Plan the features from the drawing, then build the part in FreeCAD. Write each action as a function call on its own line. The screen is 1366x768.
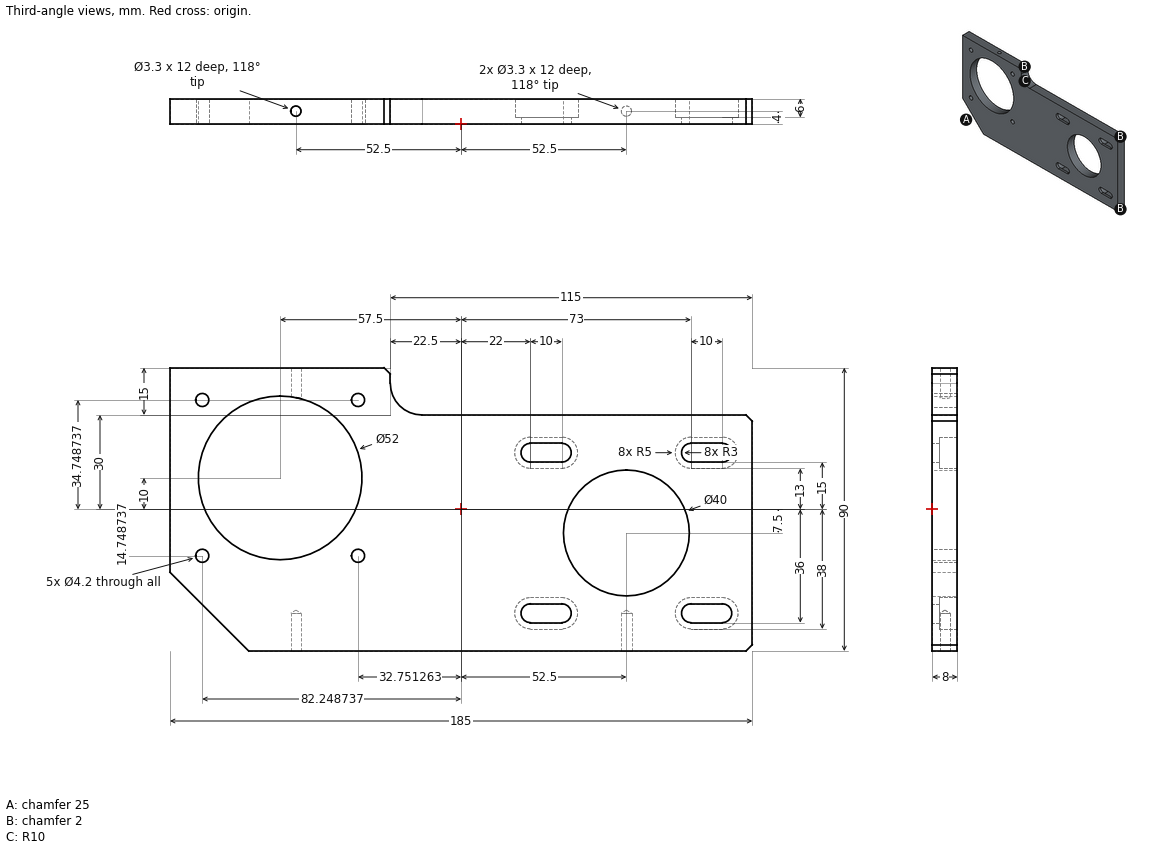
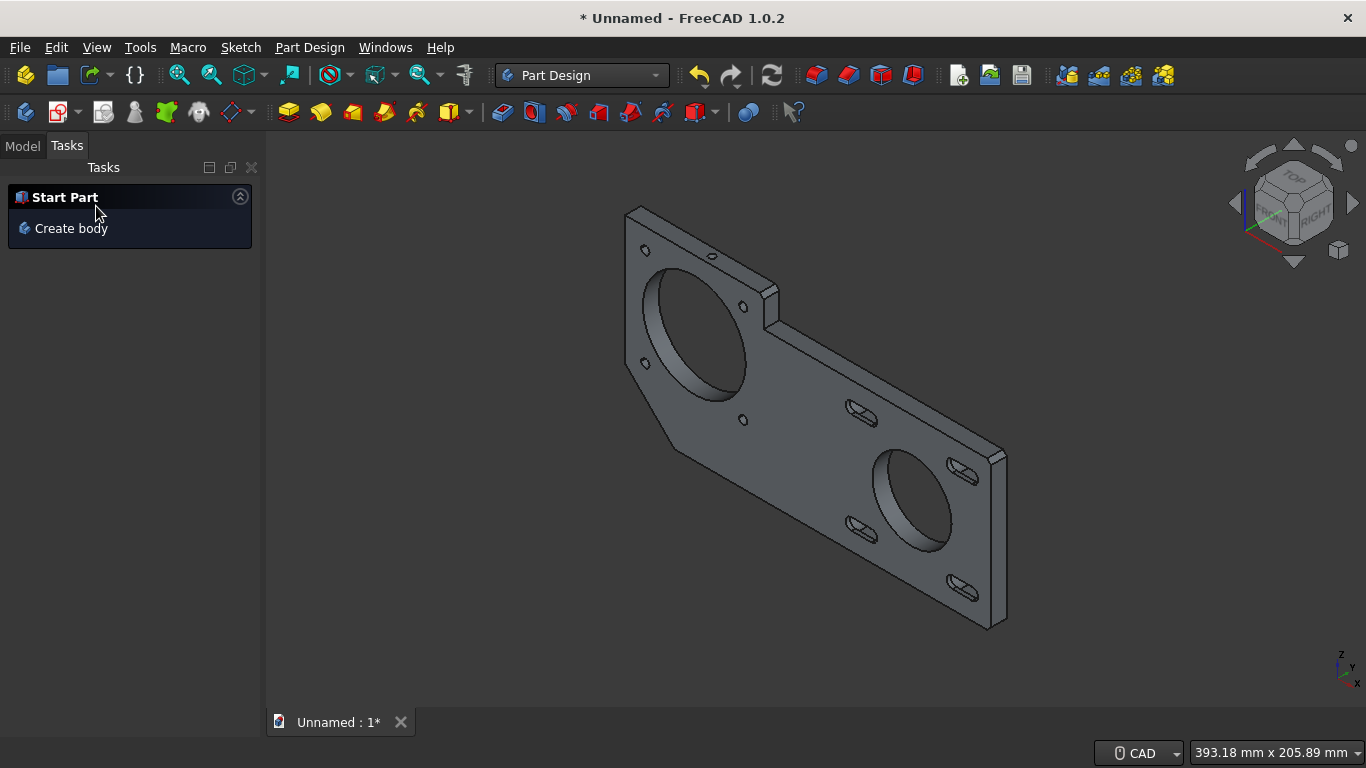
key(2)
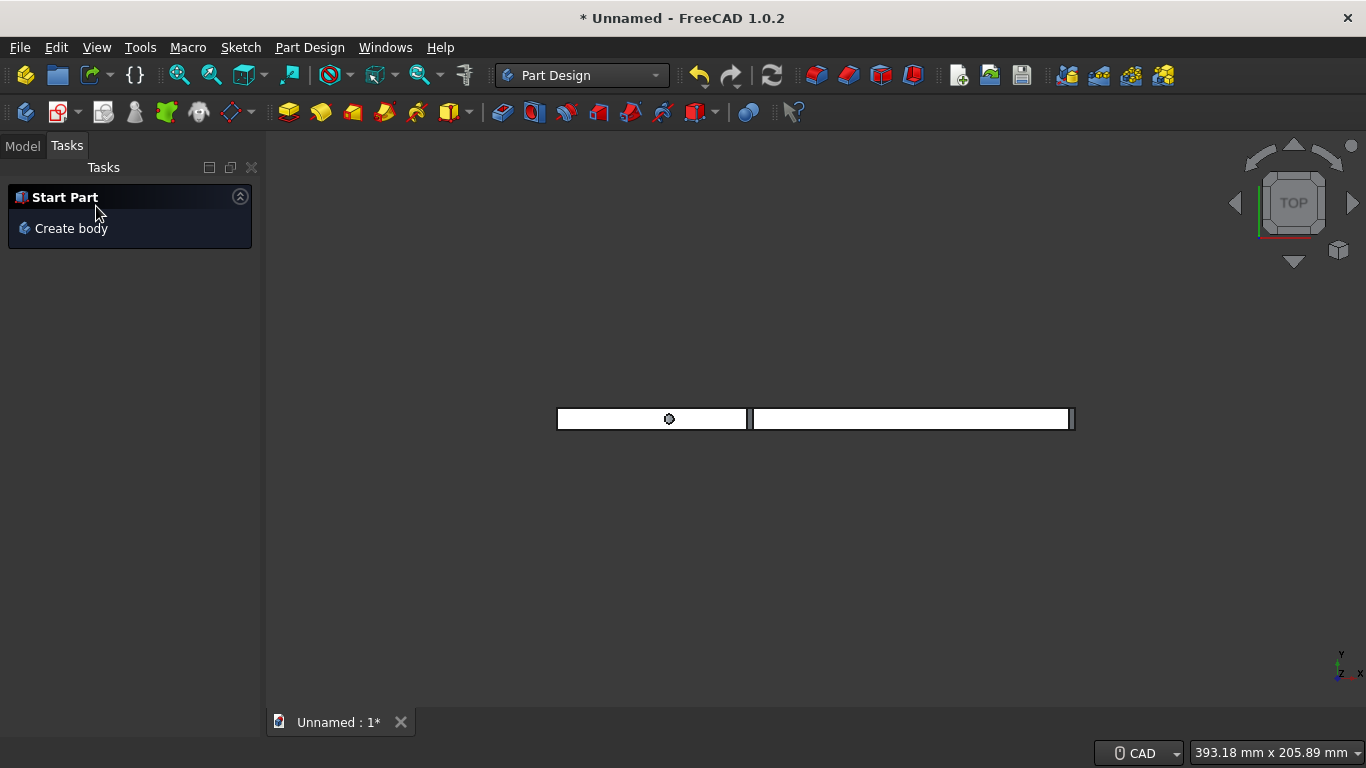
key(0)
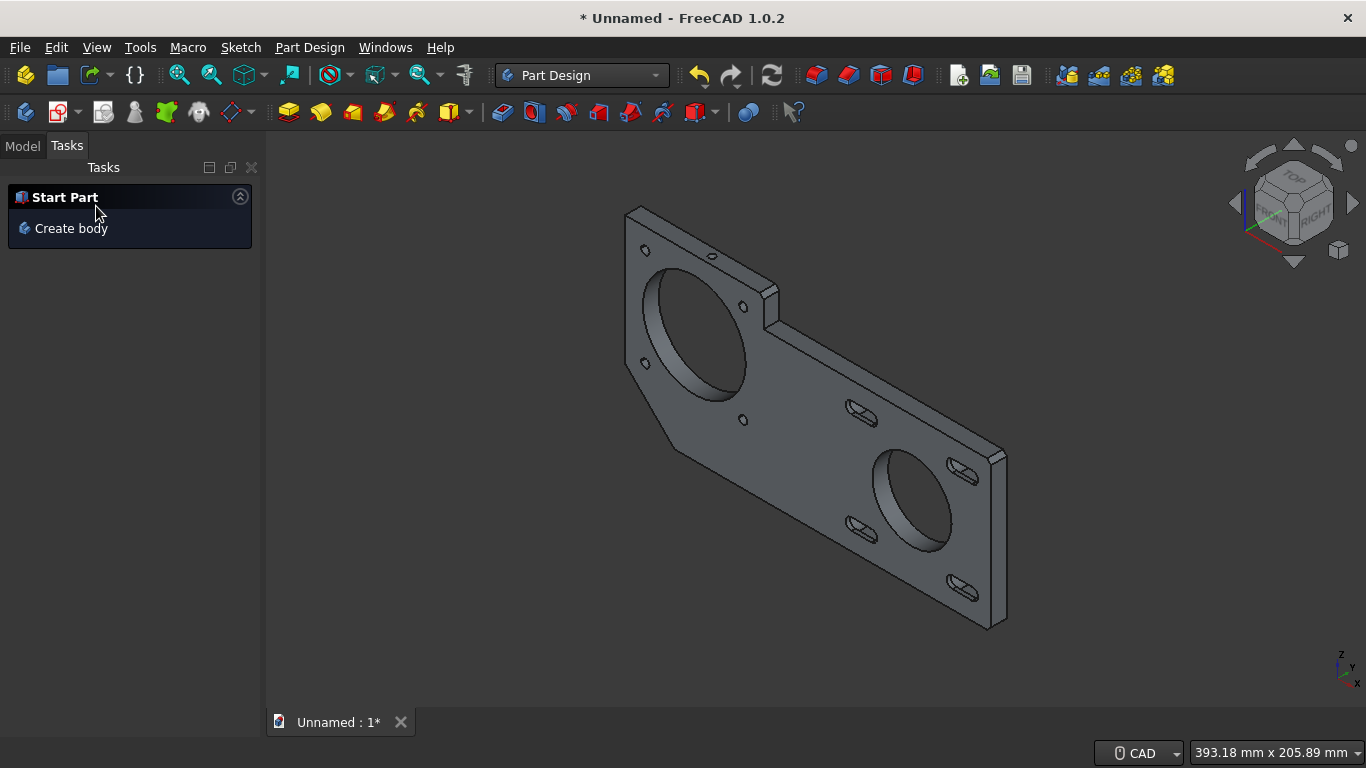
key(1)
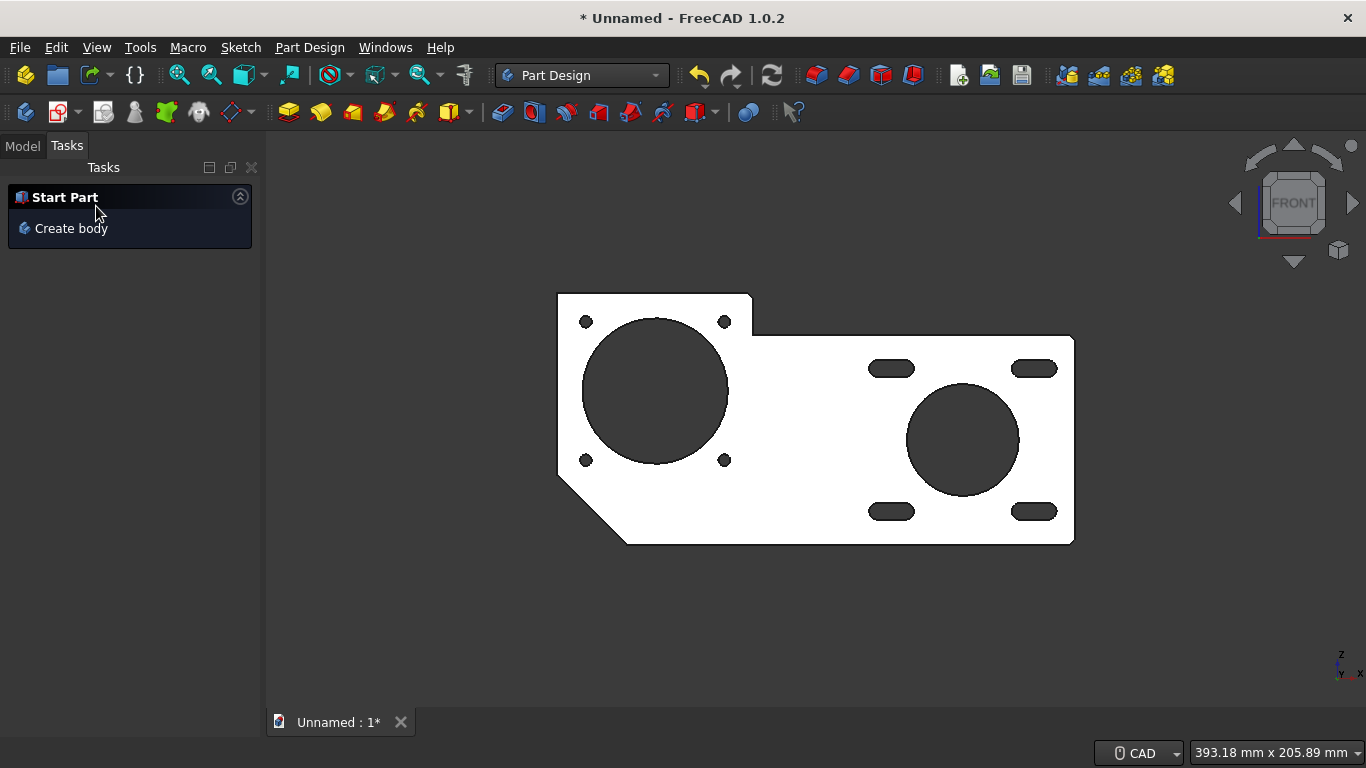
key(3)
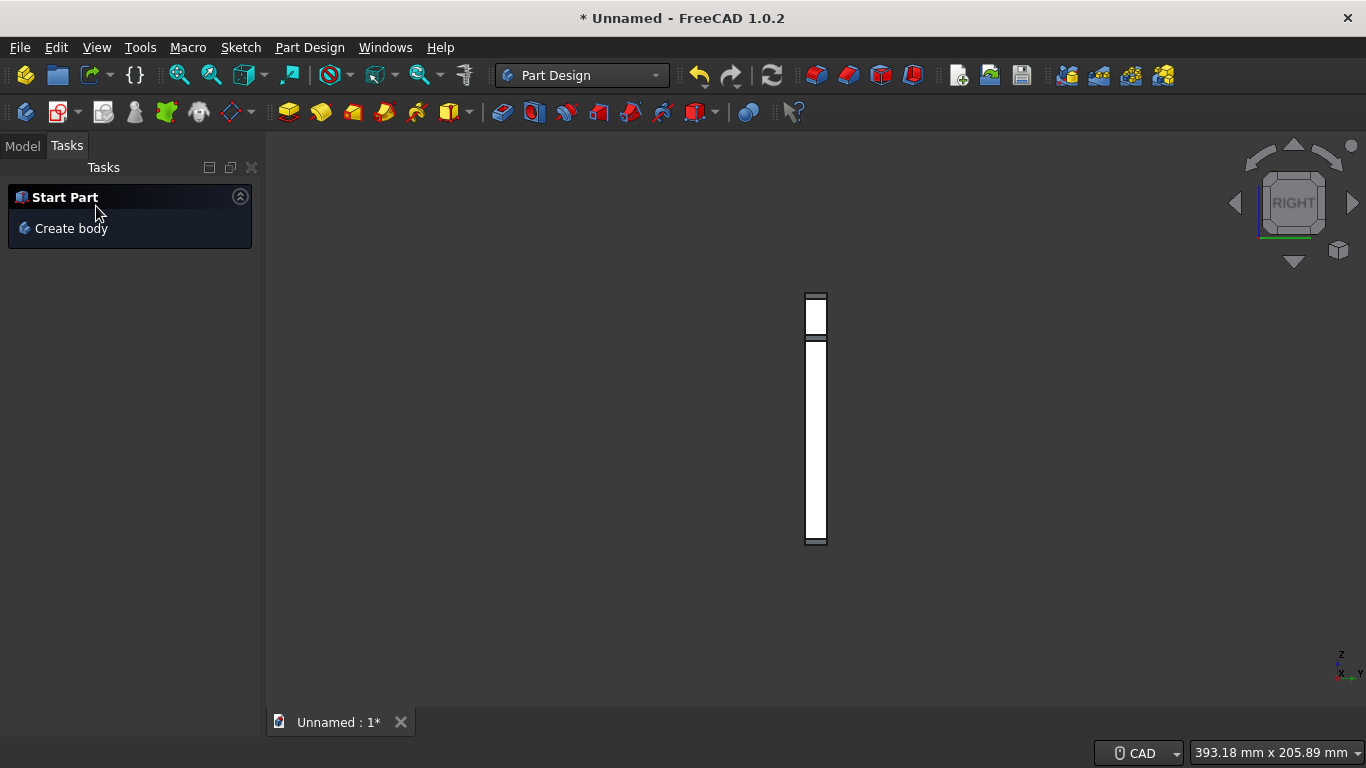
click(180, 76)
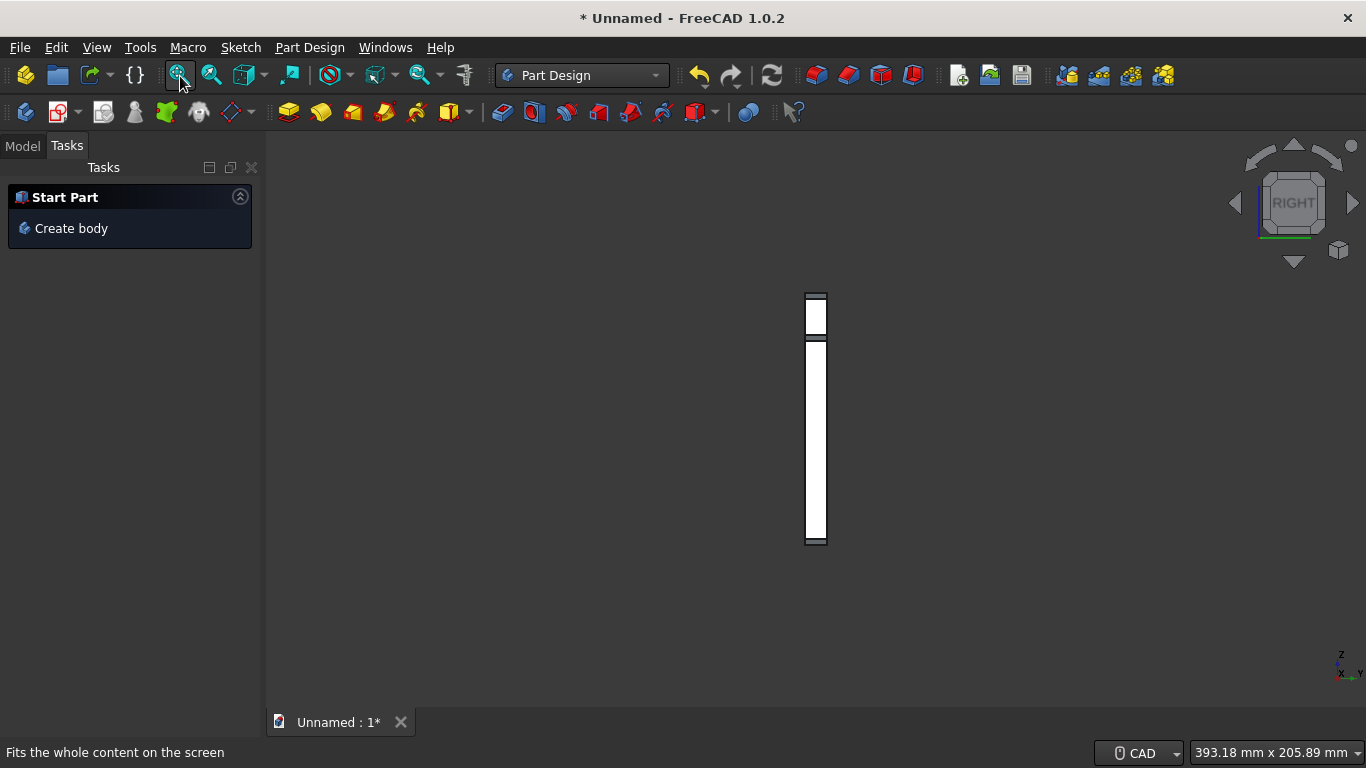
key(5)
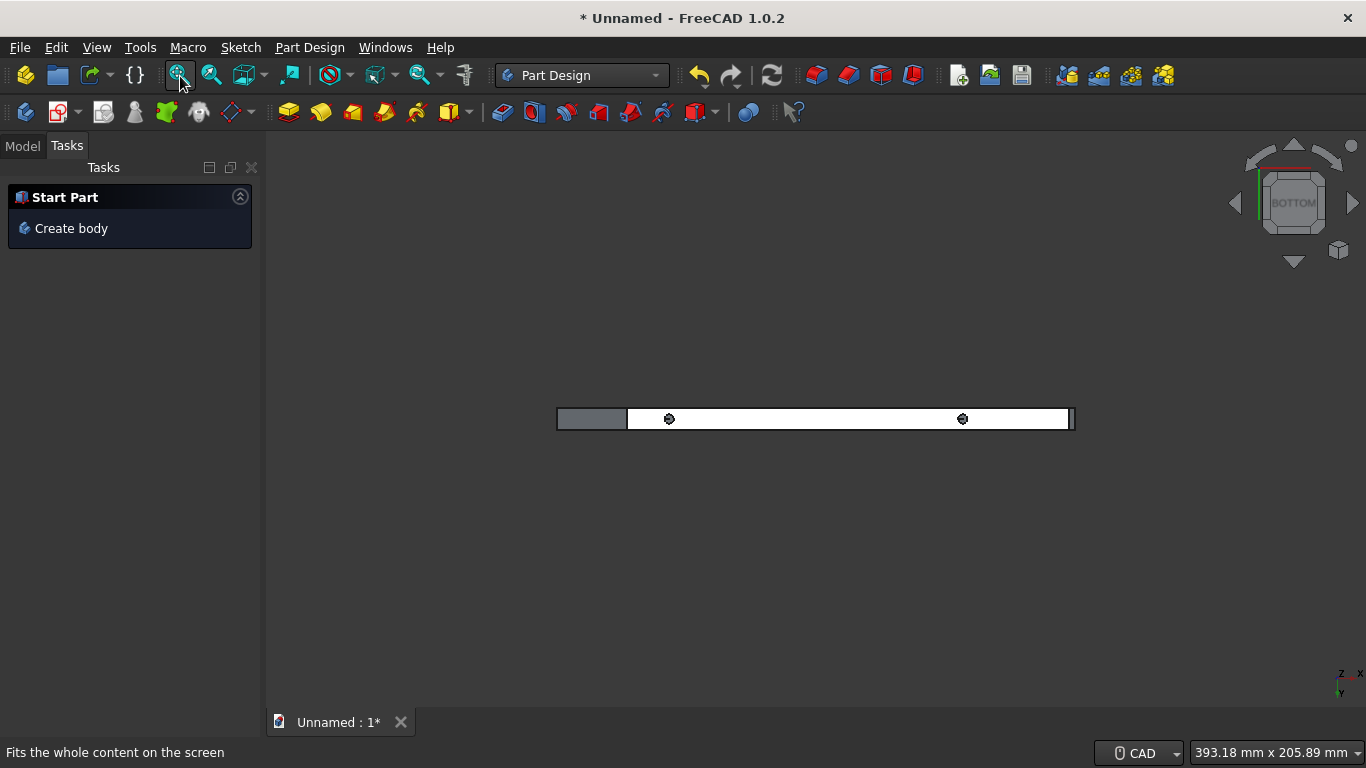
key(4)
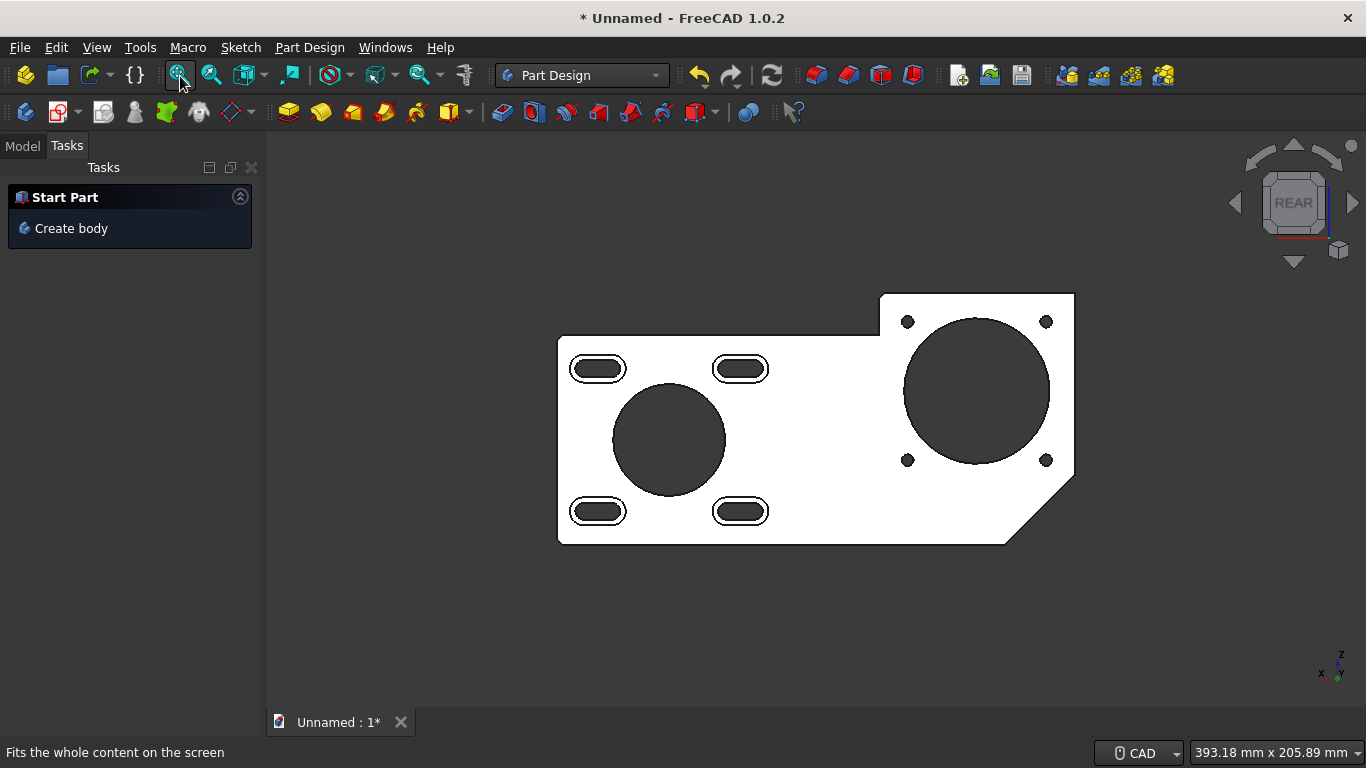
key(6)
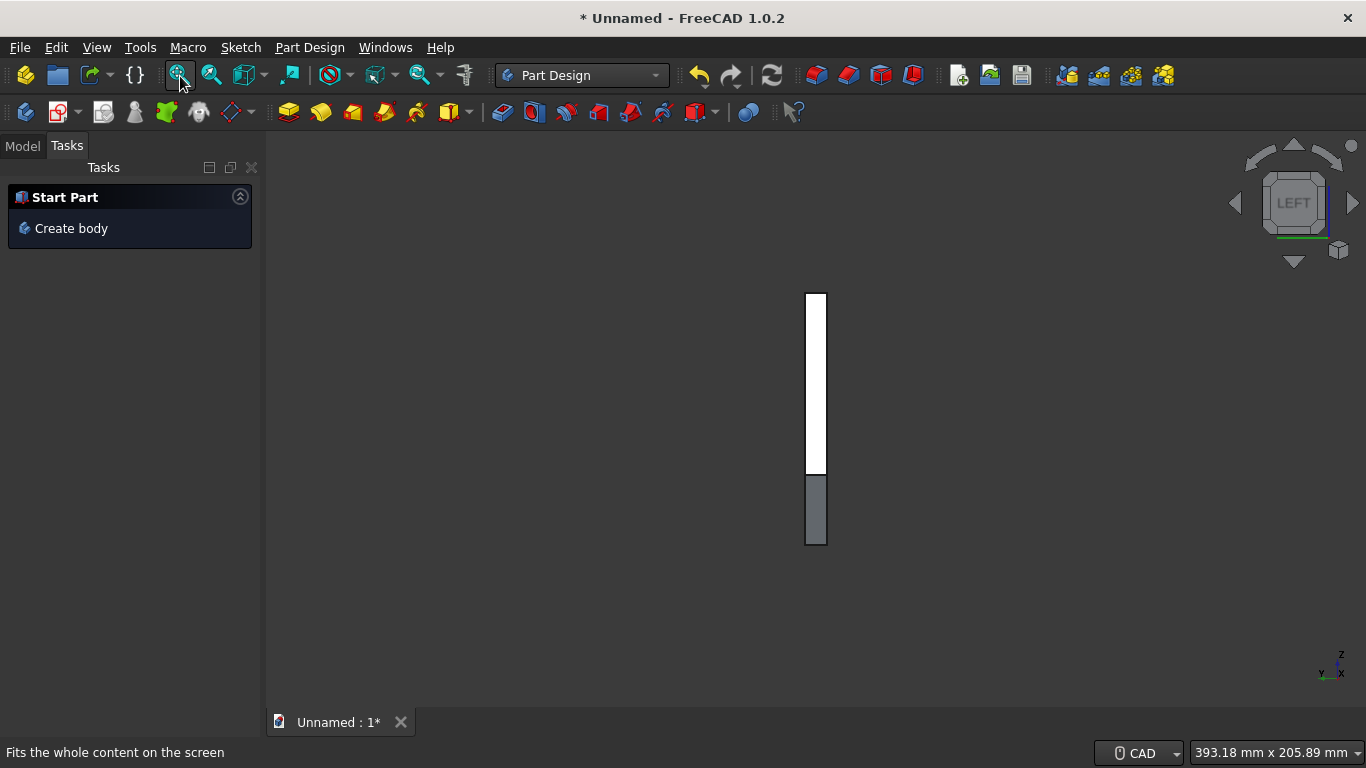
key(v)
key(f)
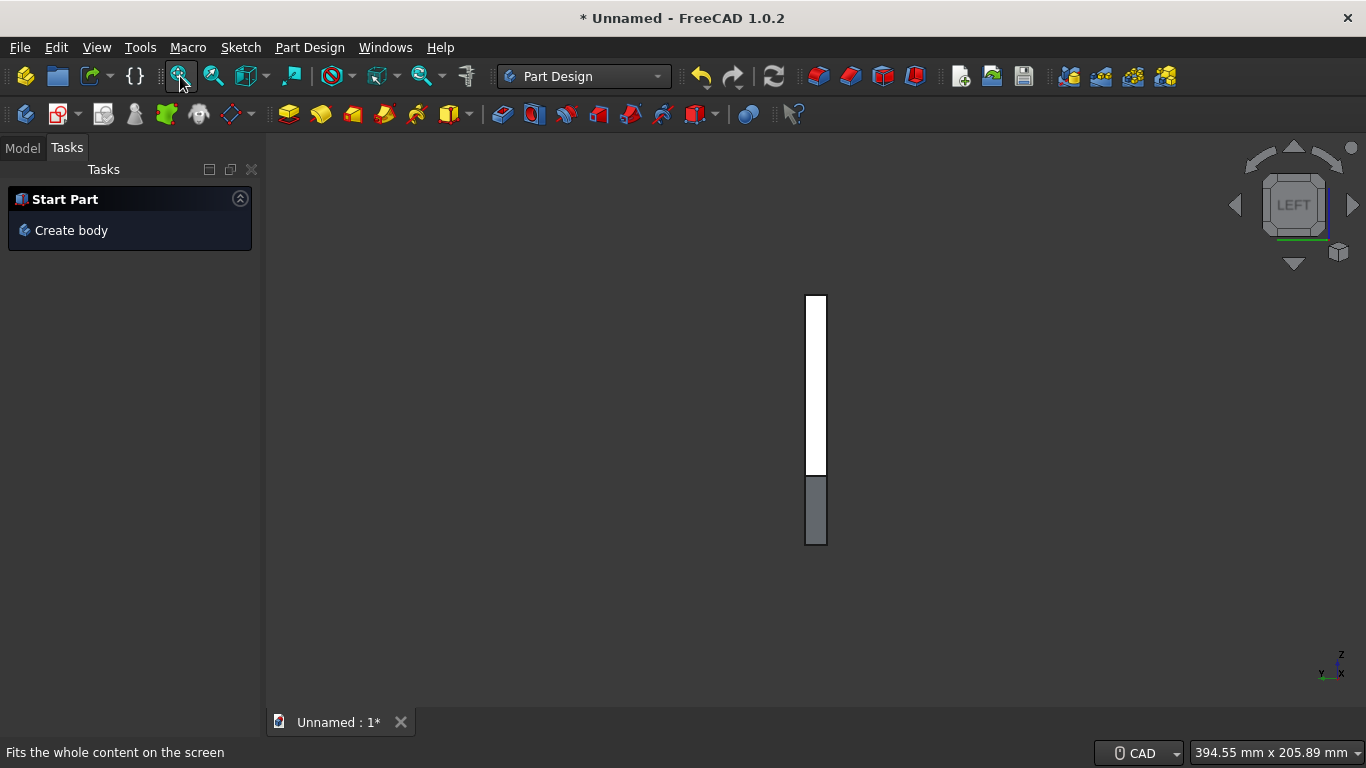
key(v)
key(3)